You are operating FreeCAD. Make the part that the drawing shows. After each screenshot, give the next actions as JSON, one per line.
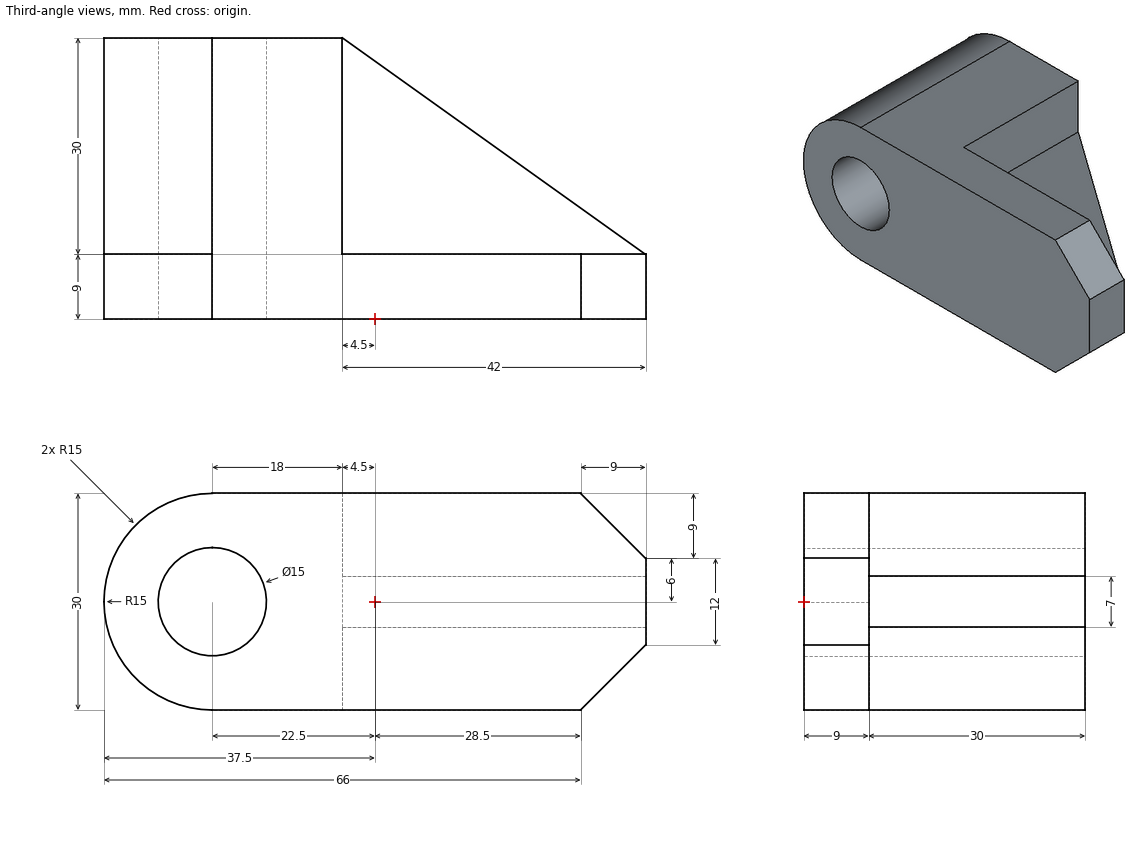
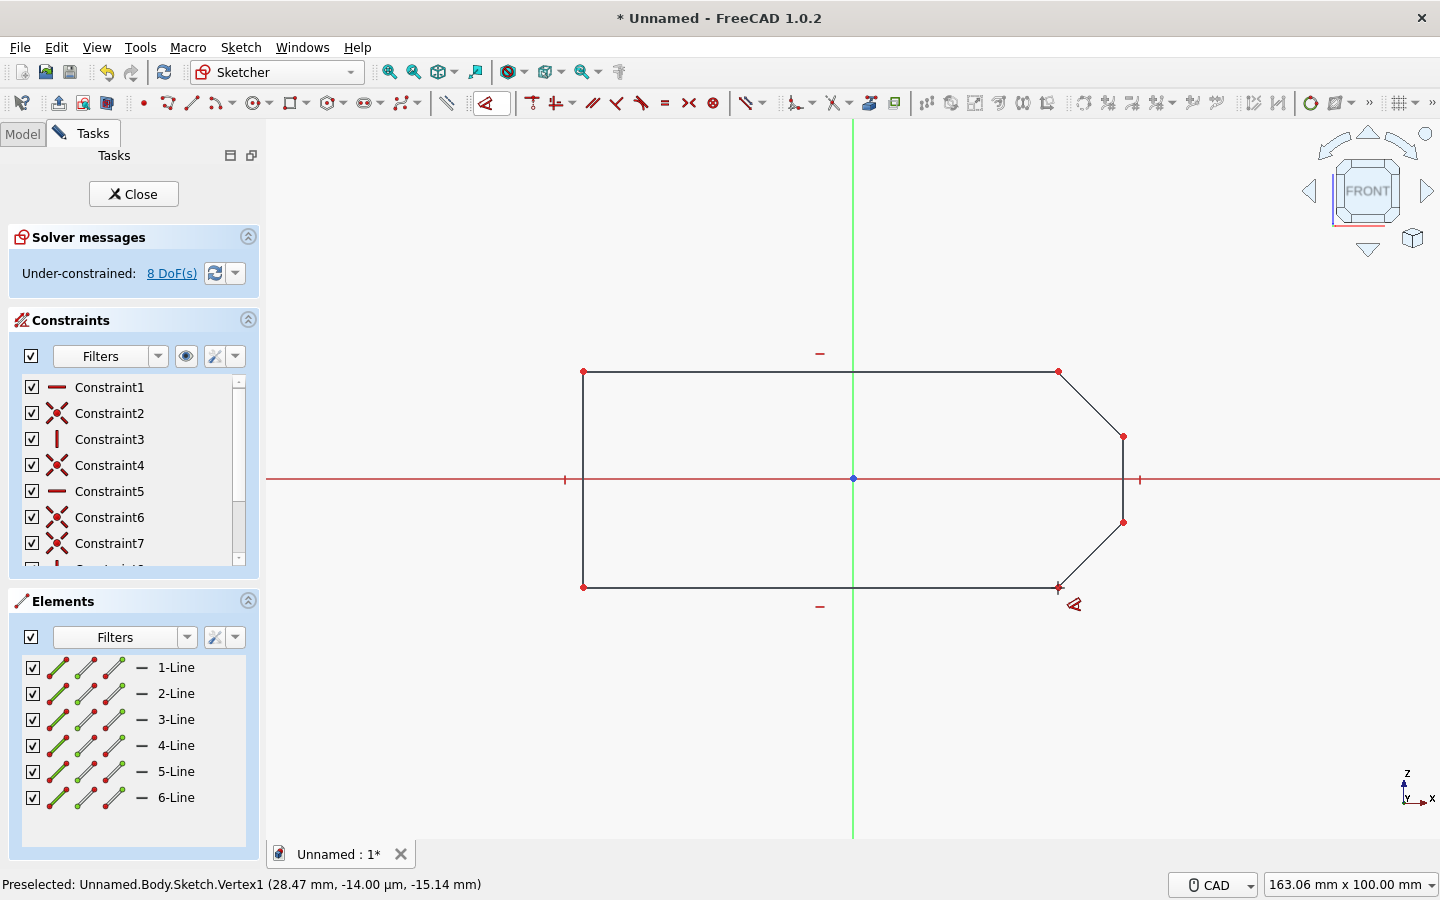
{"action": "left_click", "coordinate": [915, 588]}
{"action": "left_click", "coordinate": [820, 622]}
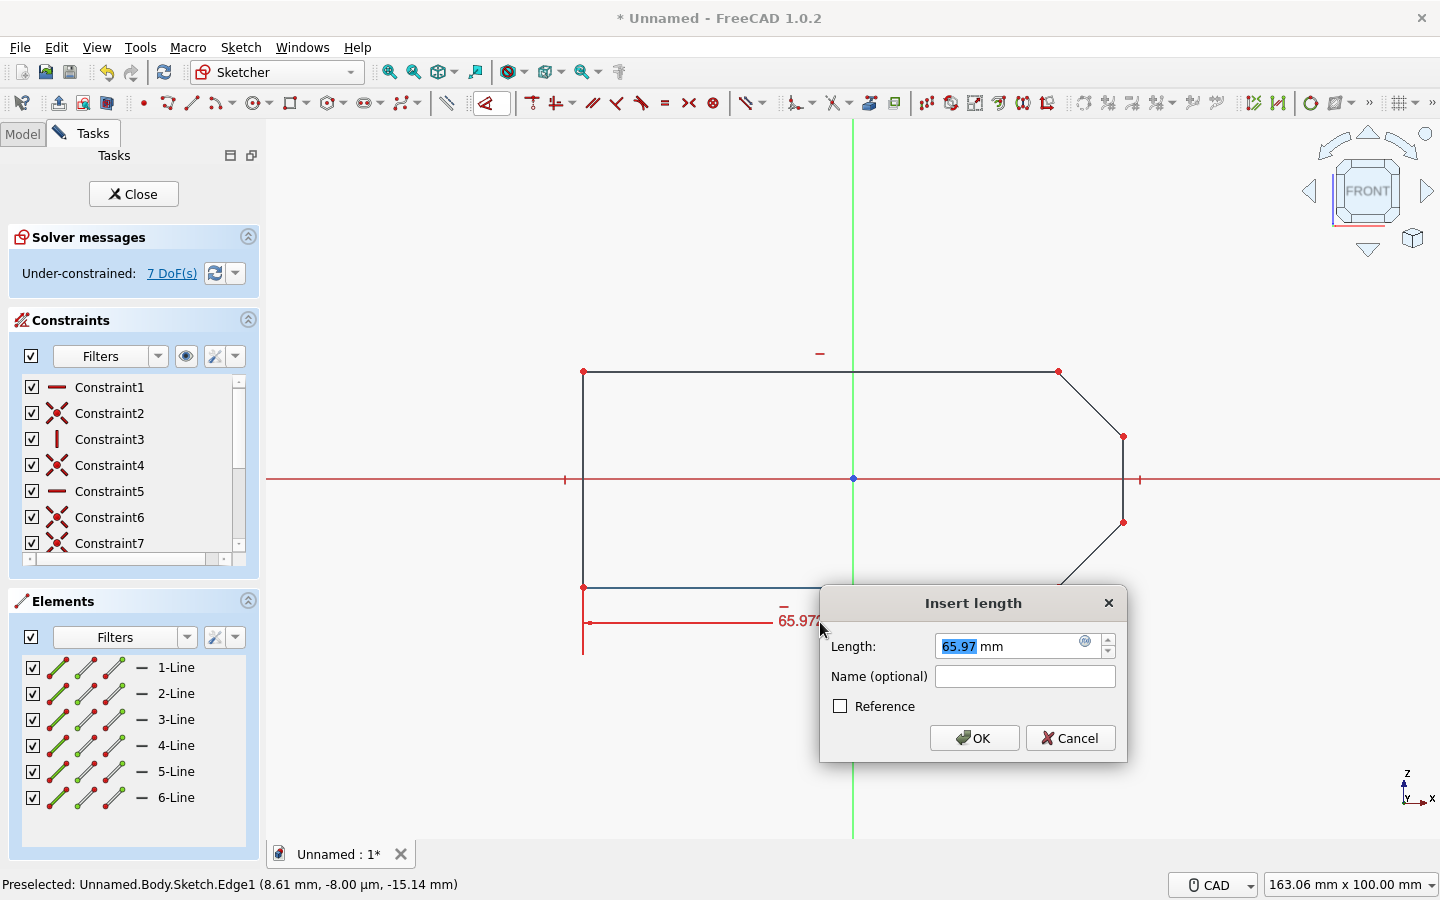
{"action": "type", "text": "66"}
{"action": "key", "text": "Return"}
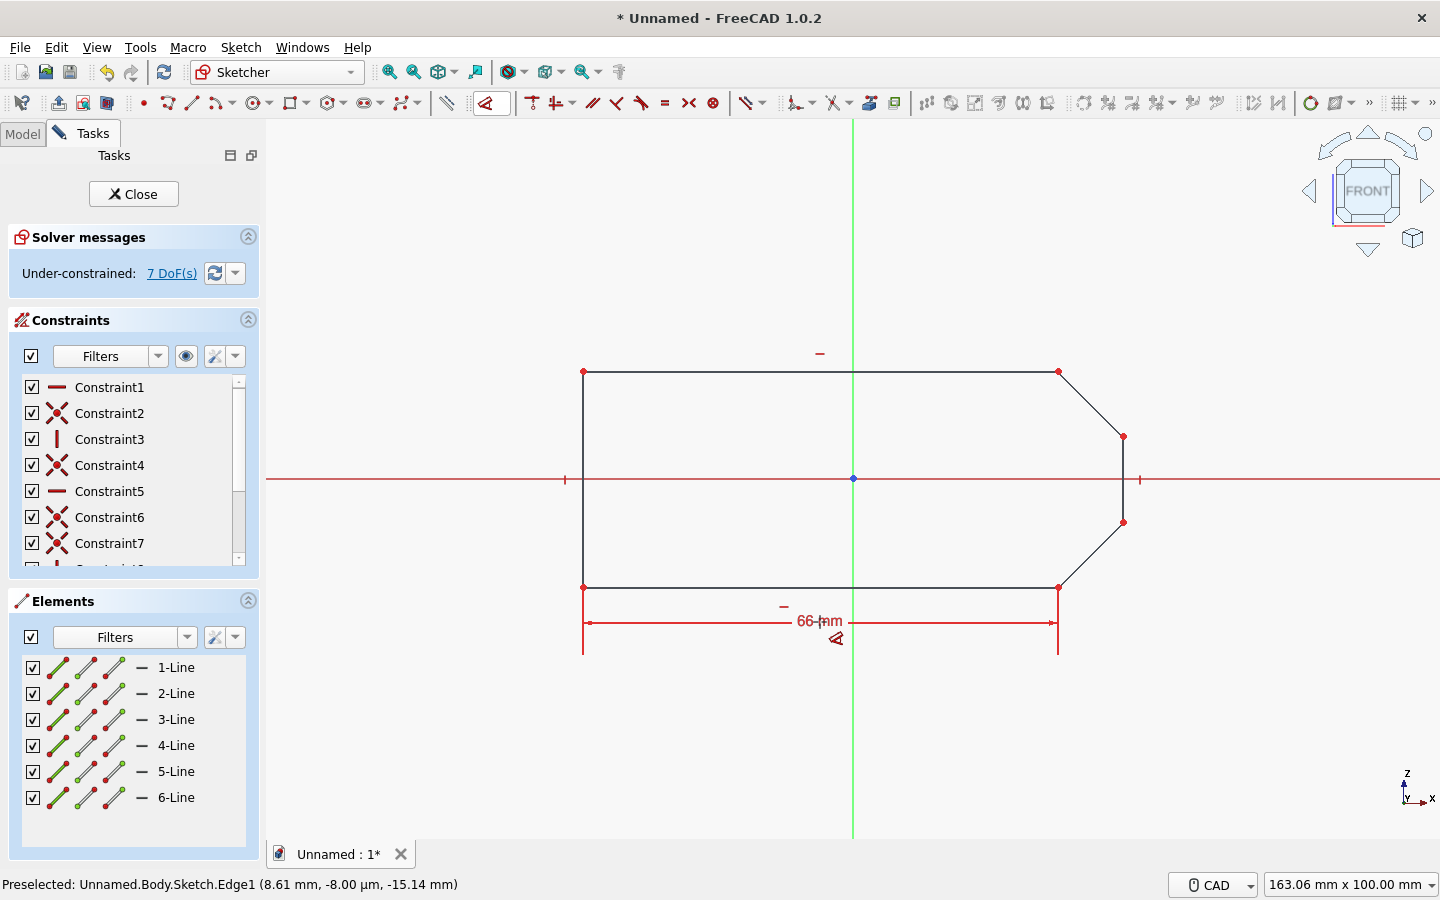
{"action": "left_click", "coordinate": [583, 523]}
{"action": "left_click", "coordinate": [549, 430]}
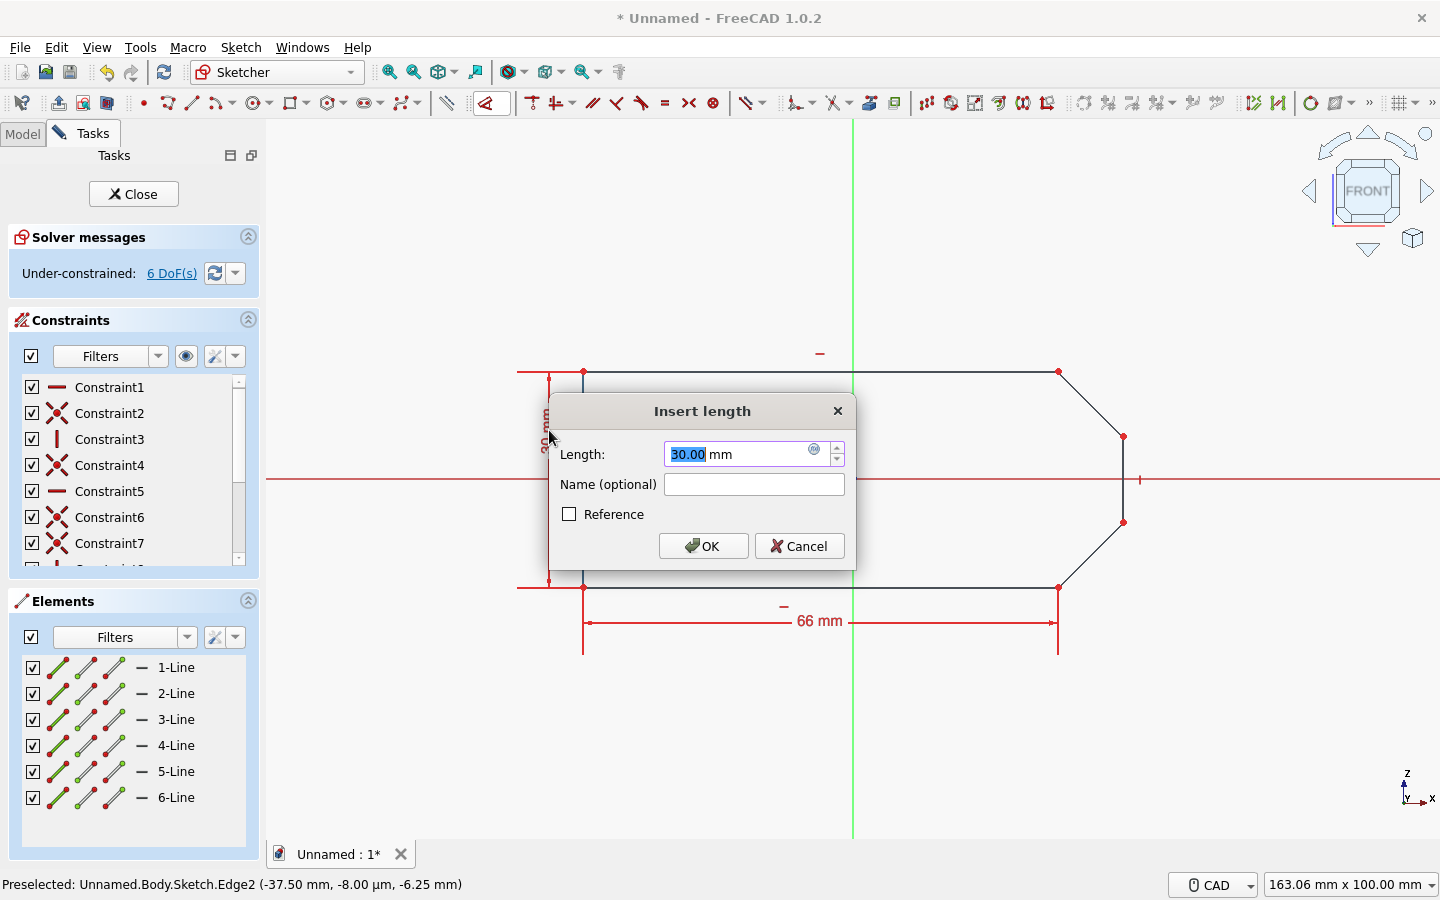
{"action": "type", "text": "30"}
{"action": "key", "text": "Return"}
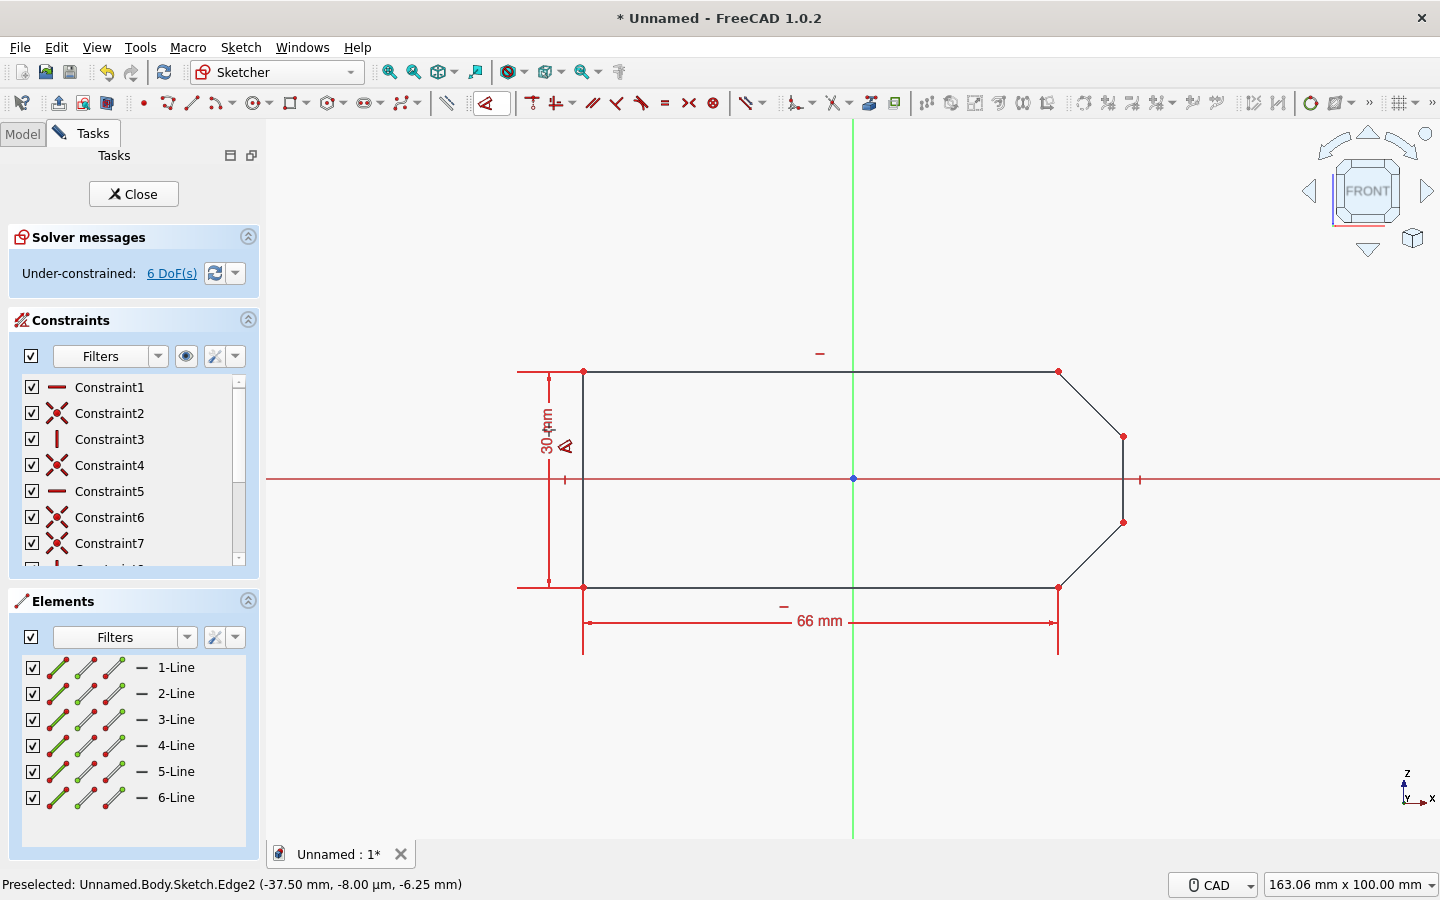
{"action": "left_click", "coordinate": [725, 372]}
{"action": "left_click", "coordinate": [820, 338]}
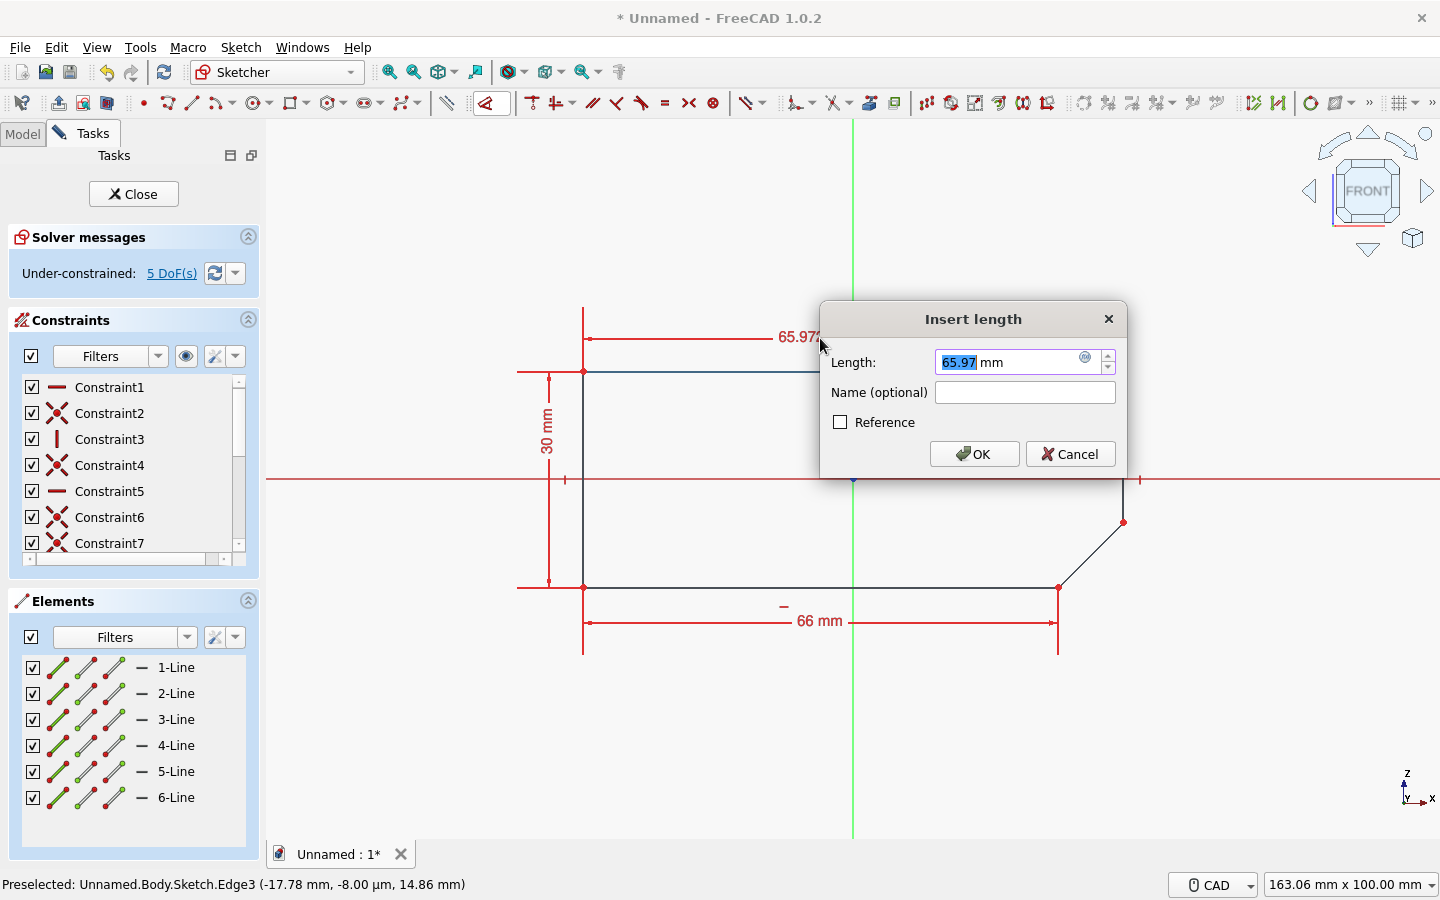
{"action": "type", "text": "66"}
{"action": "key", "text": "Return"}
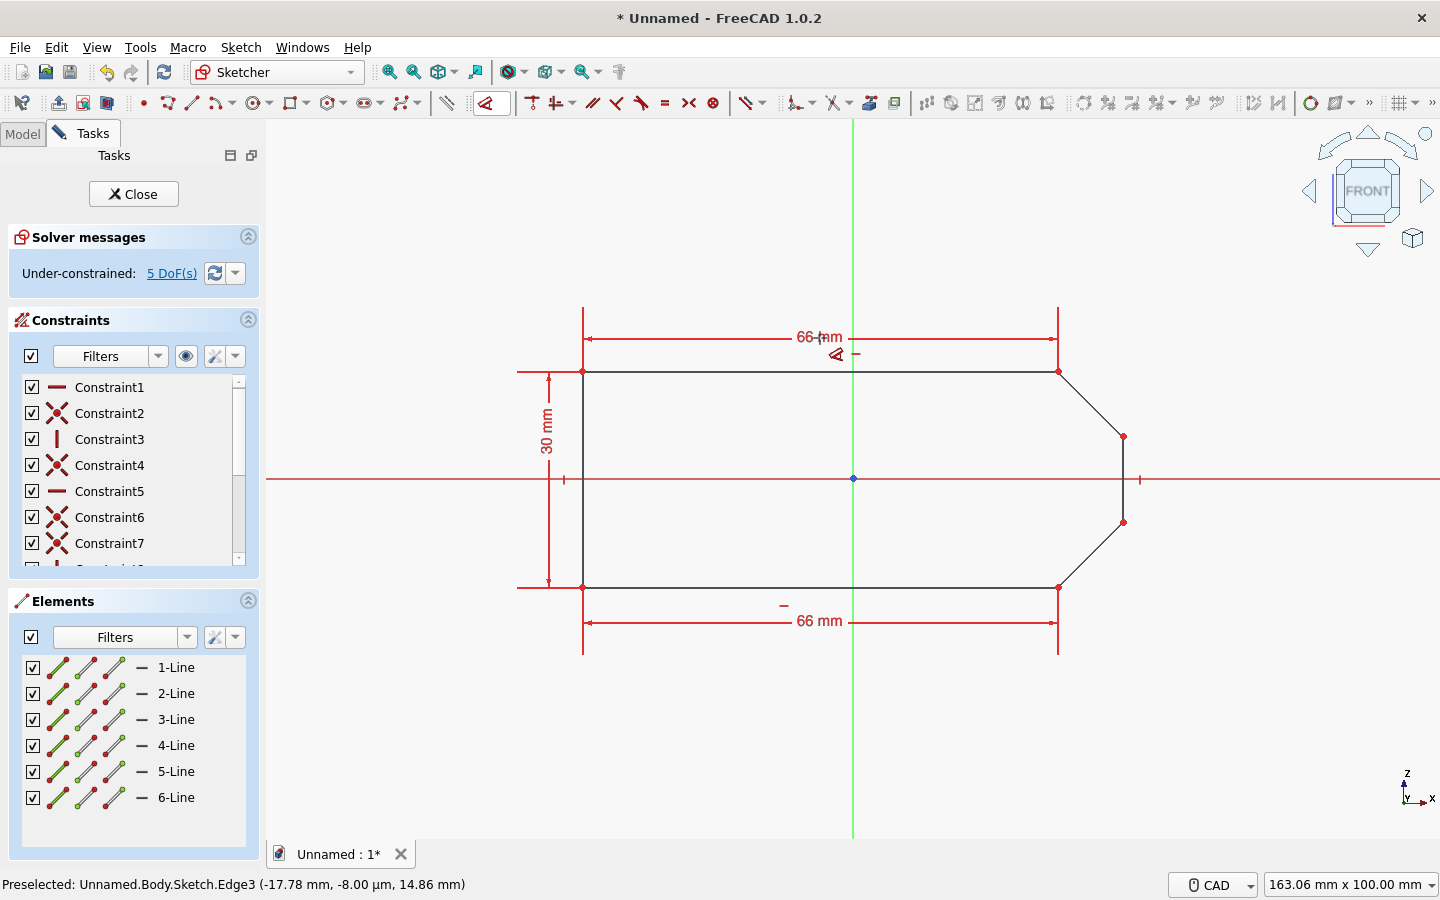
{"action": "left_click", "coordinate": [1123, 463]}
{"action": "left_click", "coordinate": [1157, 460]}